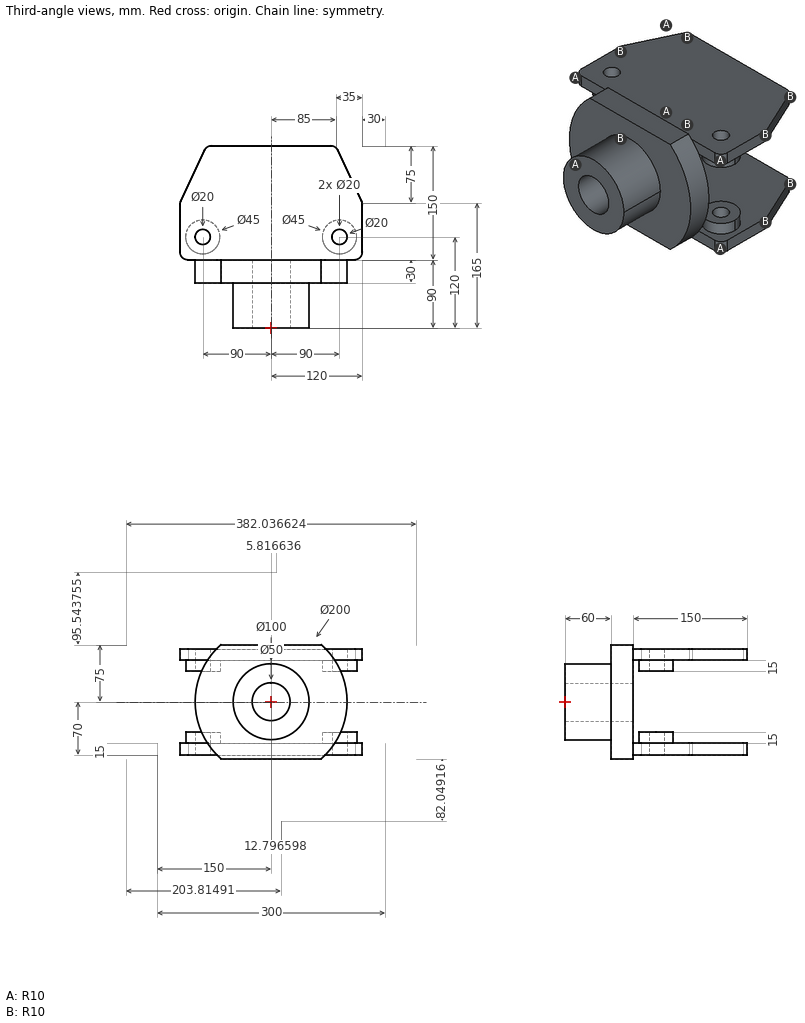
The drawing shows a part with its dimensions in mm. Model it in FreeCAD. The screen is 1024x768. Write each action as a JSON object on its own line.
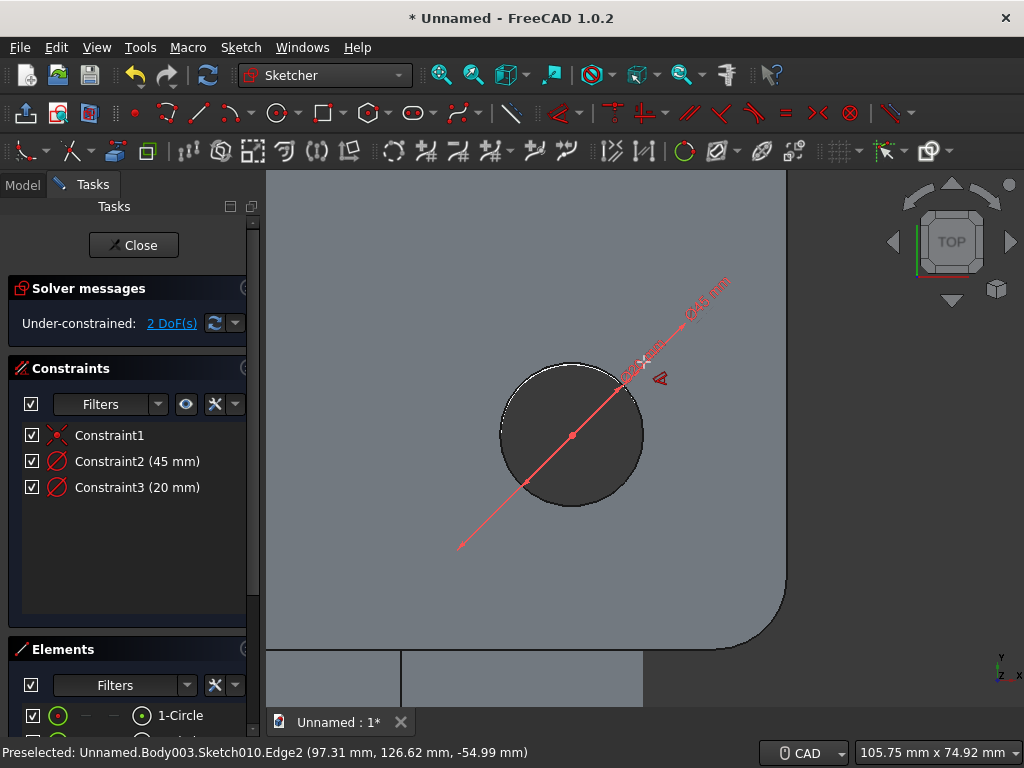
{"action": "left_click", "coordinate": [572, 436]}
{"action": "left_click", "coordinate": [433, 402]}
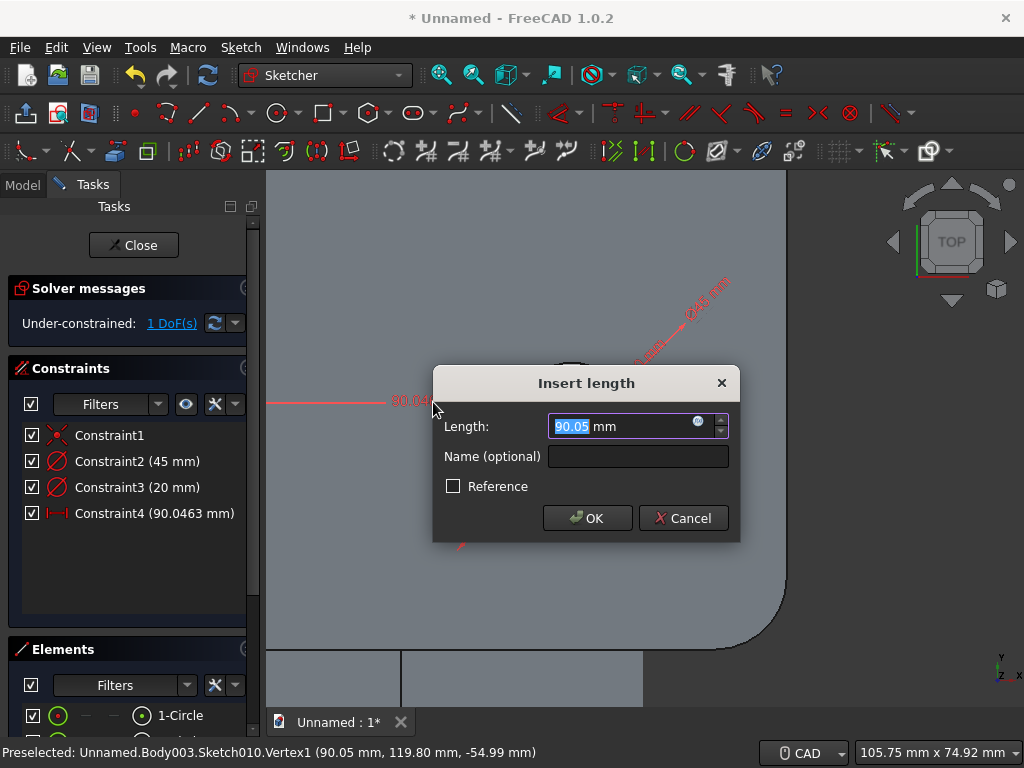
{"action": "type", "text": "90"}
{"action": "key", "text": "Return"}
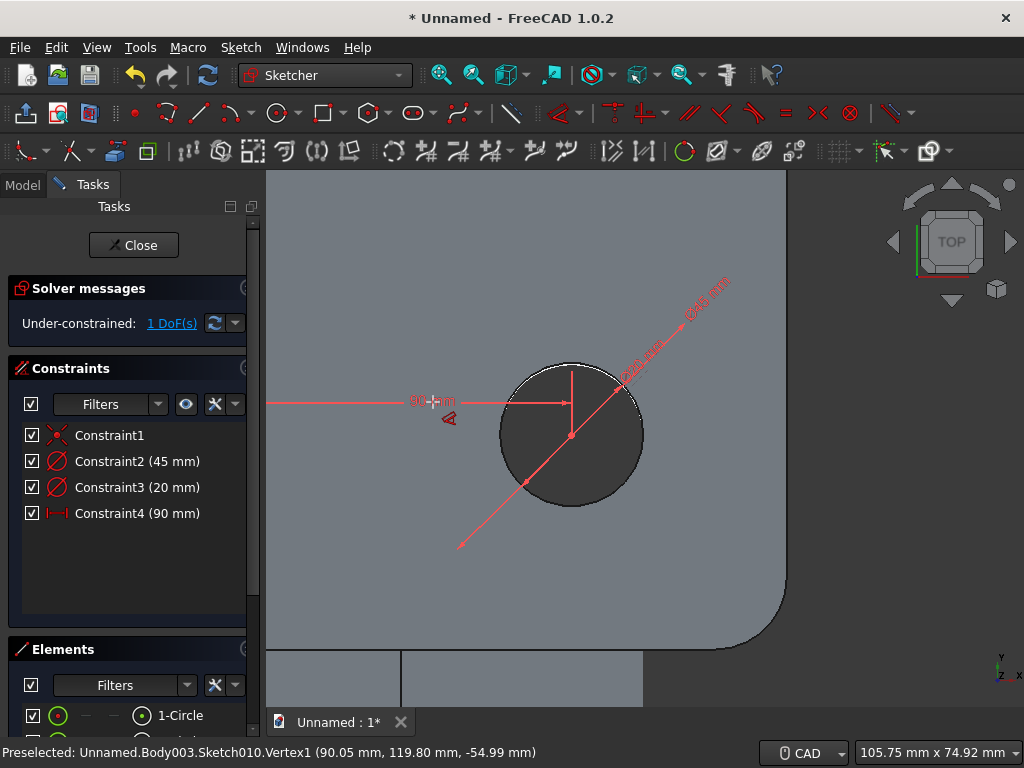
{"action": "left_click", "coordinate": [572, 436]}
{"action": "left_click", "coordinate": [606, 558]}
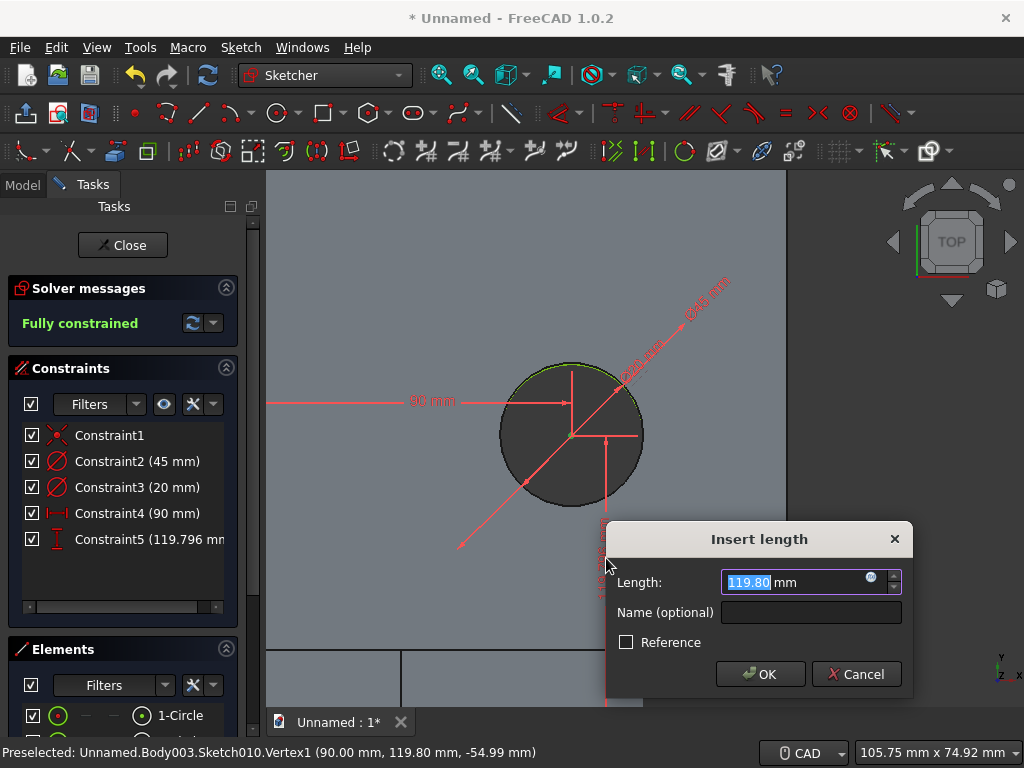
{"action": "type", "text": "120"}
{"action": "key", "text": "Return"}
{"action": "key", "text": "Escape"}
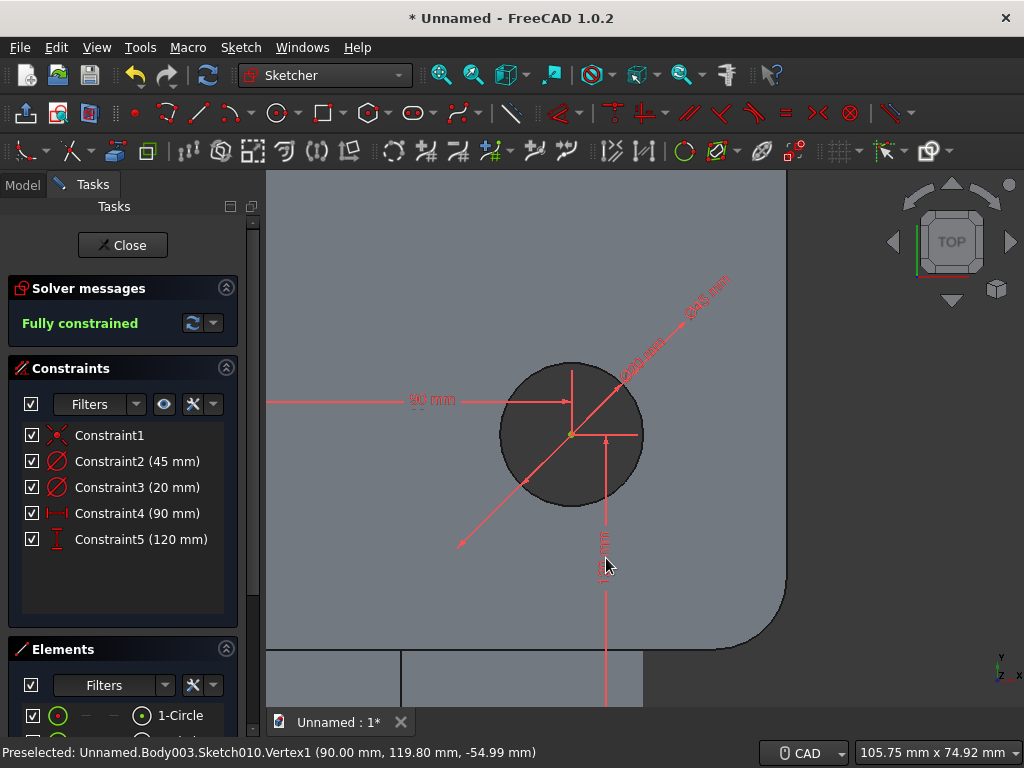
{"action": "left_click", "coordinate": [123, 245]}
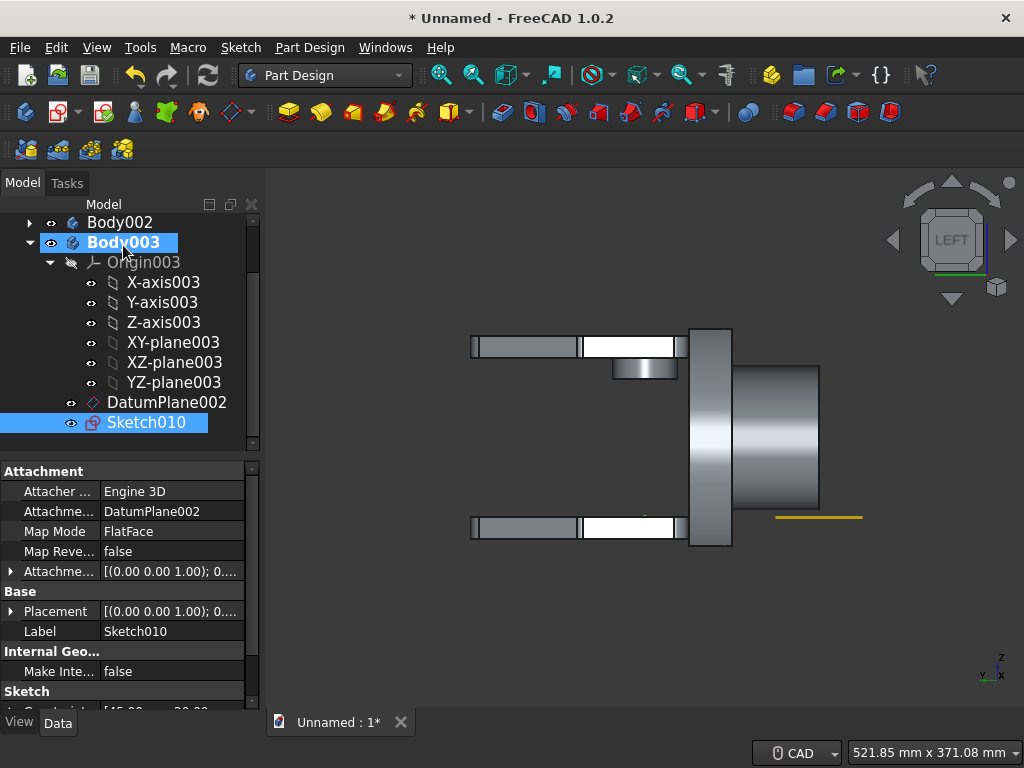
{"action": "left_click", "coordinate": [290, 112]}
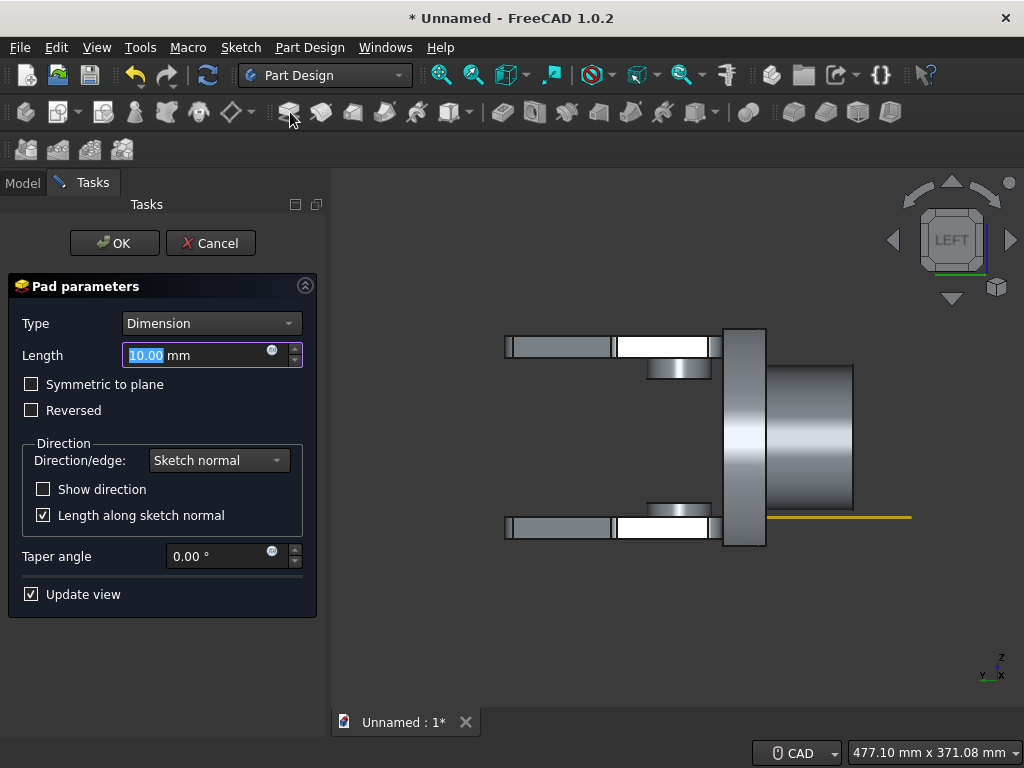
{"action": "type", "text": "15"}
{"action": "key", "text": "Tab"}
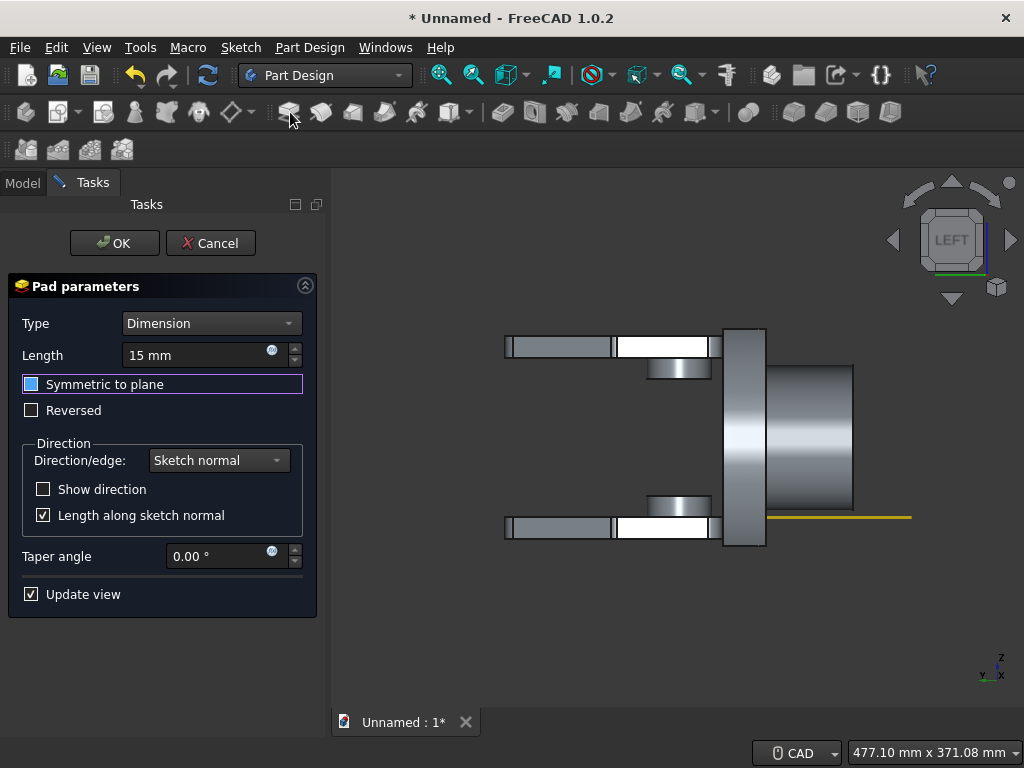
{"action": "left_click", "coordinate": [115, 243]}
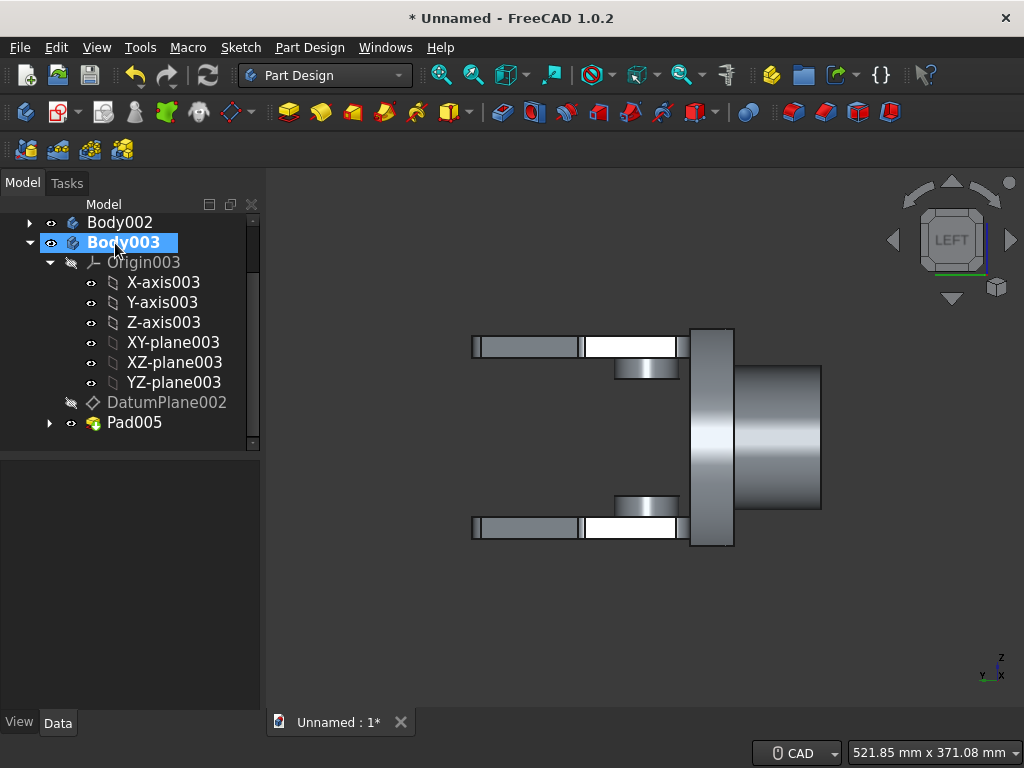
{"action": "left_click", "coordinate": [442, 76]}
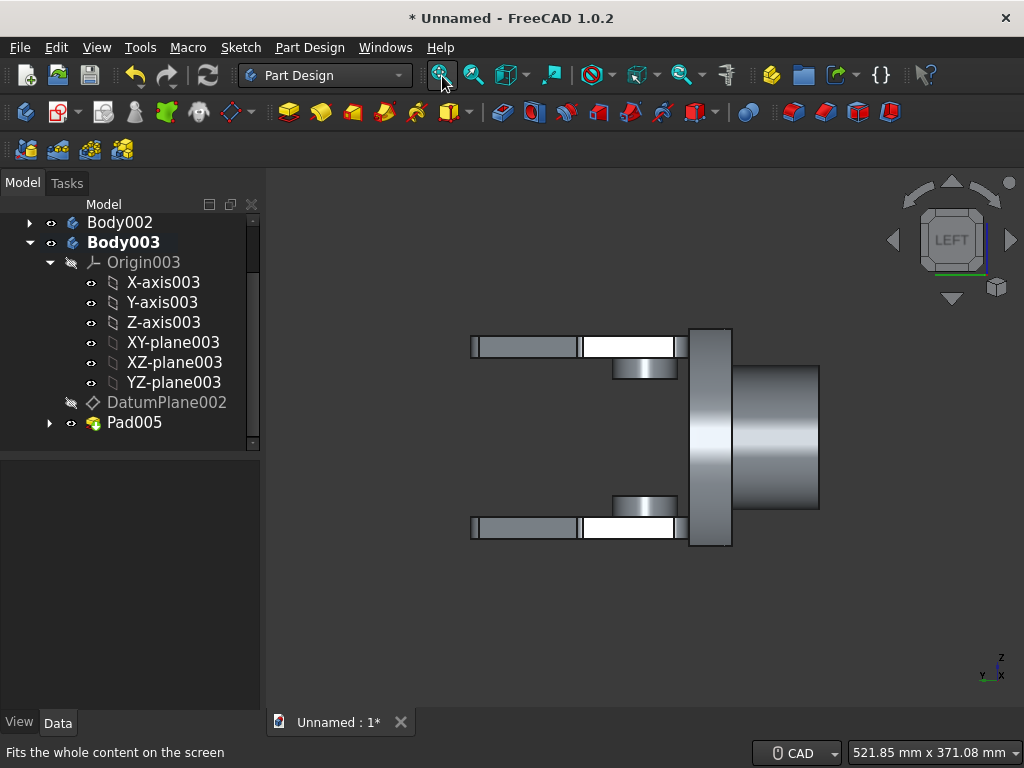
{"action": "left_click", "coordinate": [26, 112]}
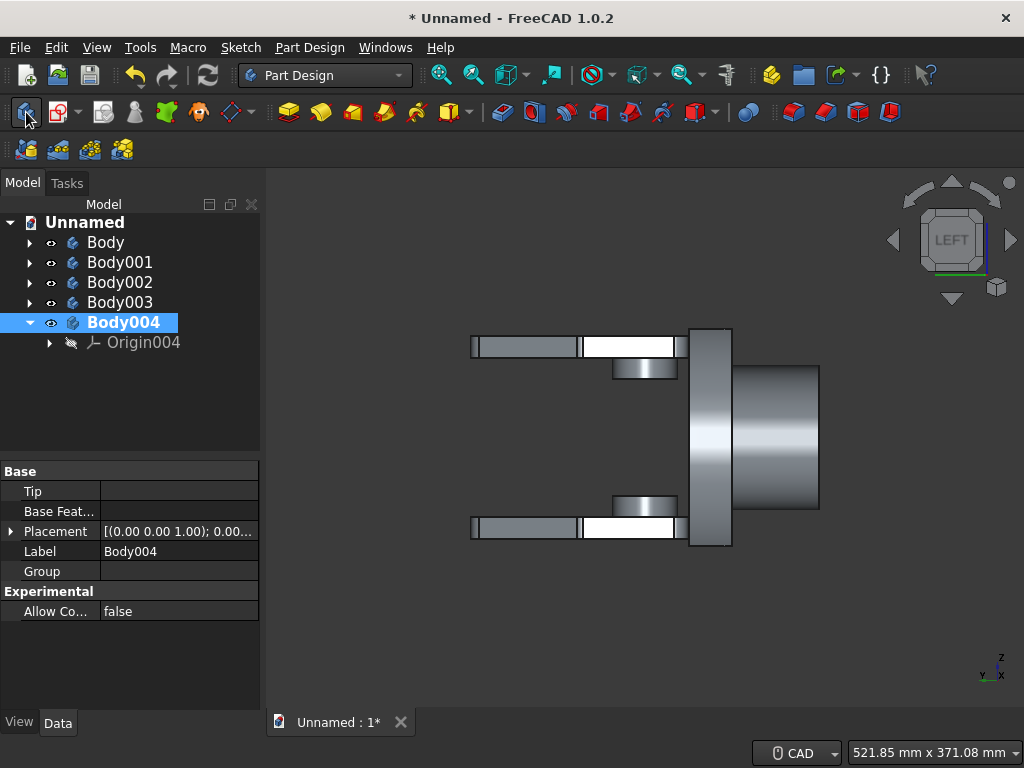
{"action": "left_click", "coordinate": [50, 343]}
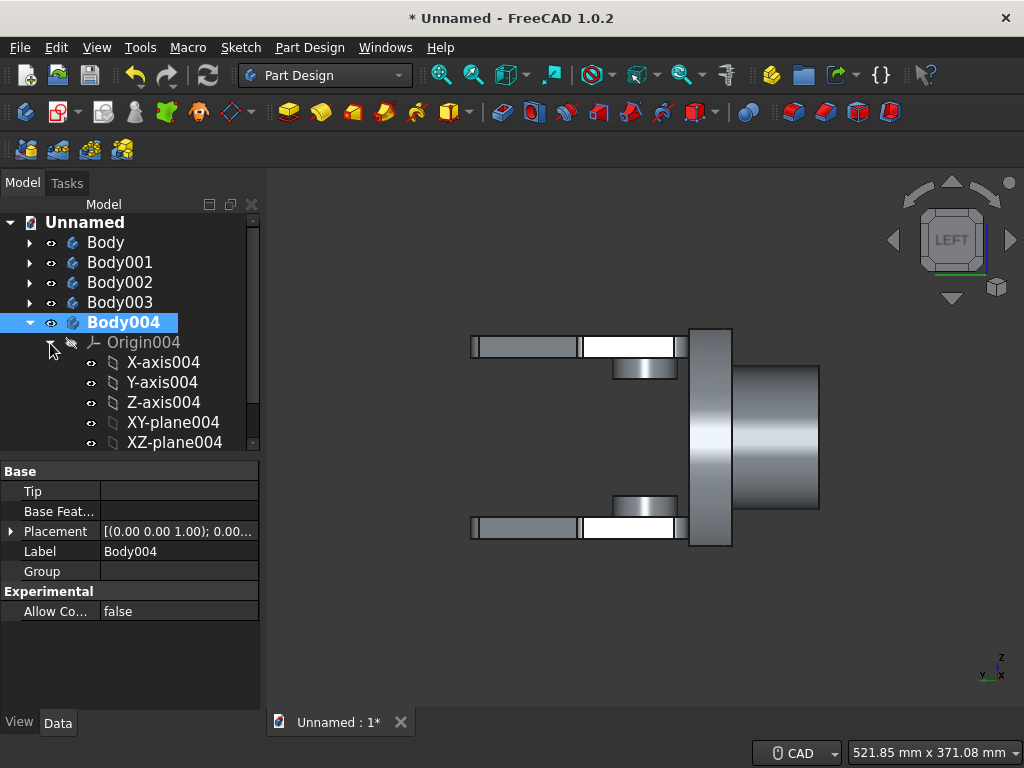
{"action": "left_click", "coordinate": [136, 423]}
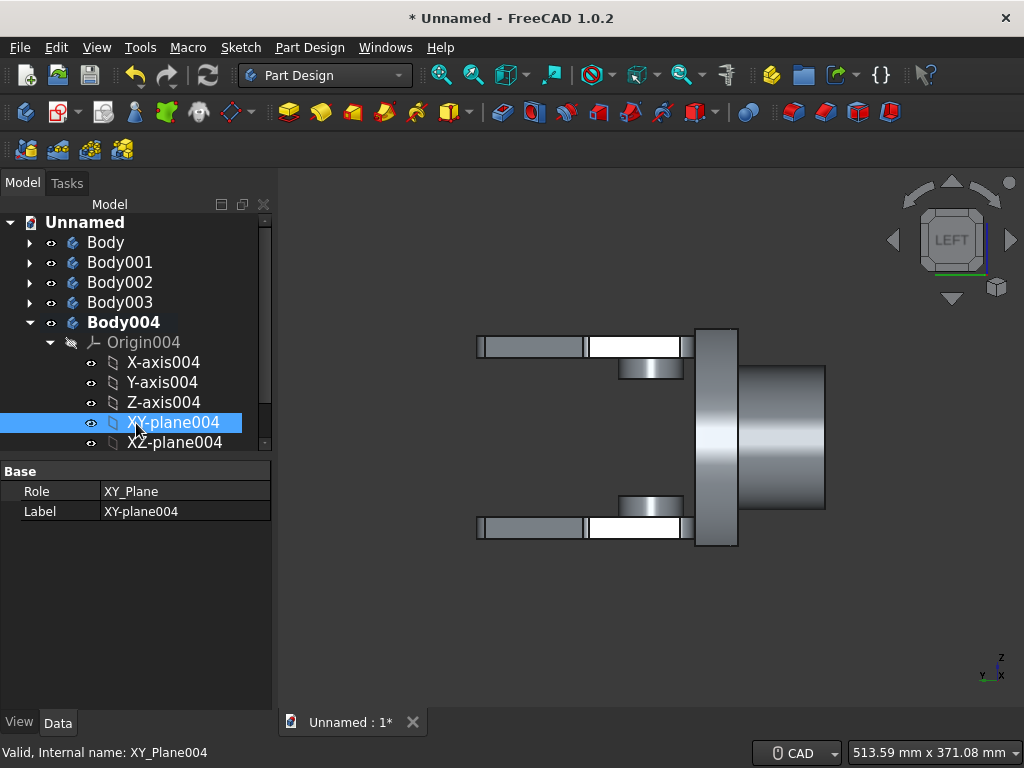
{"action": "left_click", "coordinate": [232, 112]}